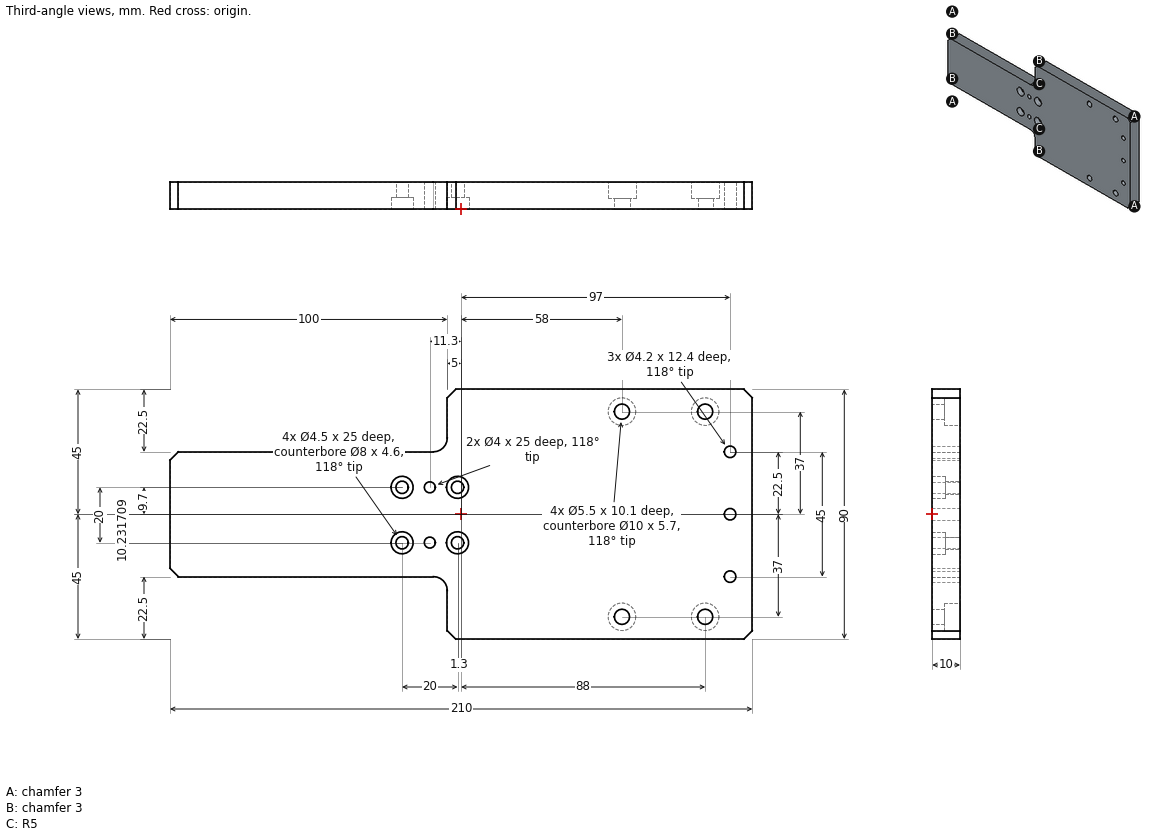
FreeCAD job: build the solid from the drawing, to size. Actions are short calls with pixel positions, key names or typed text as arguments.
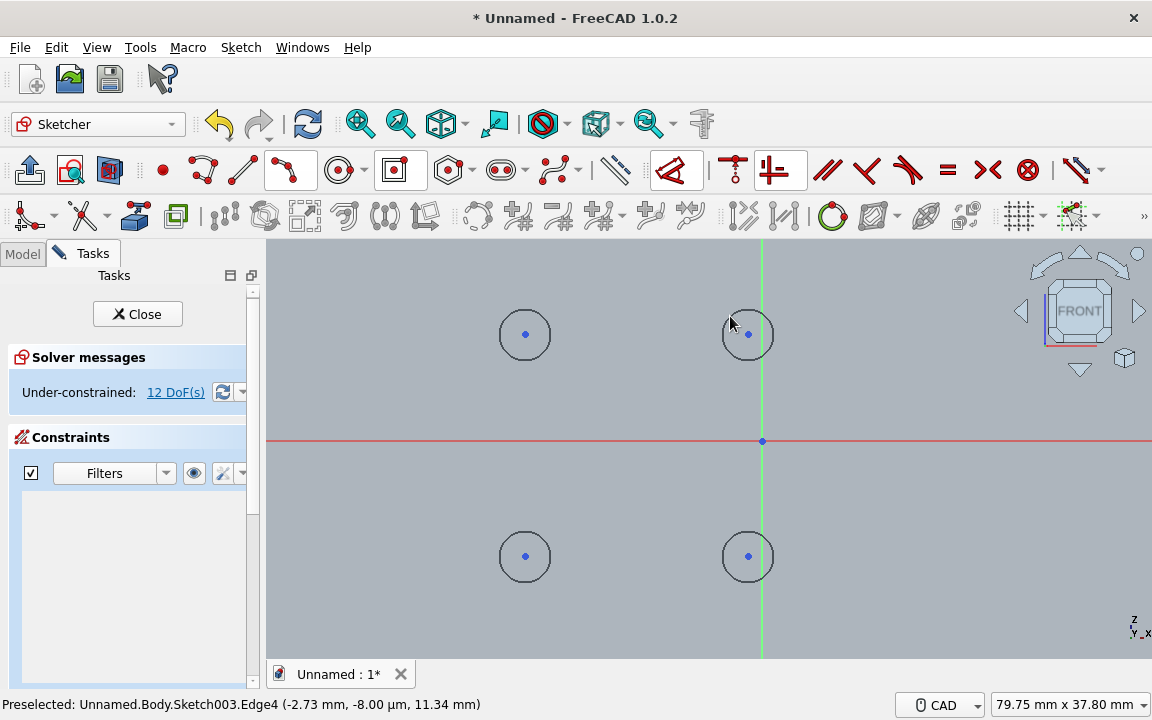
click(543, 539)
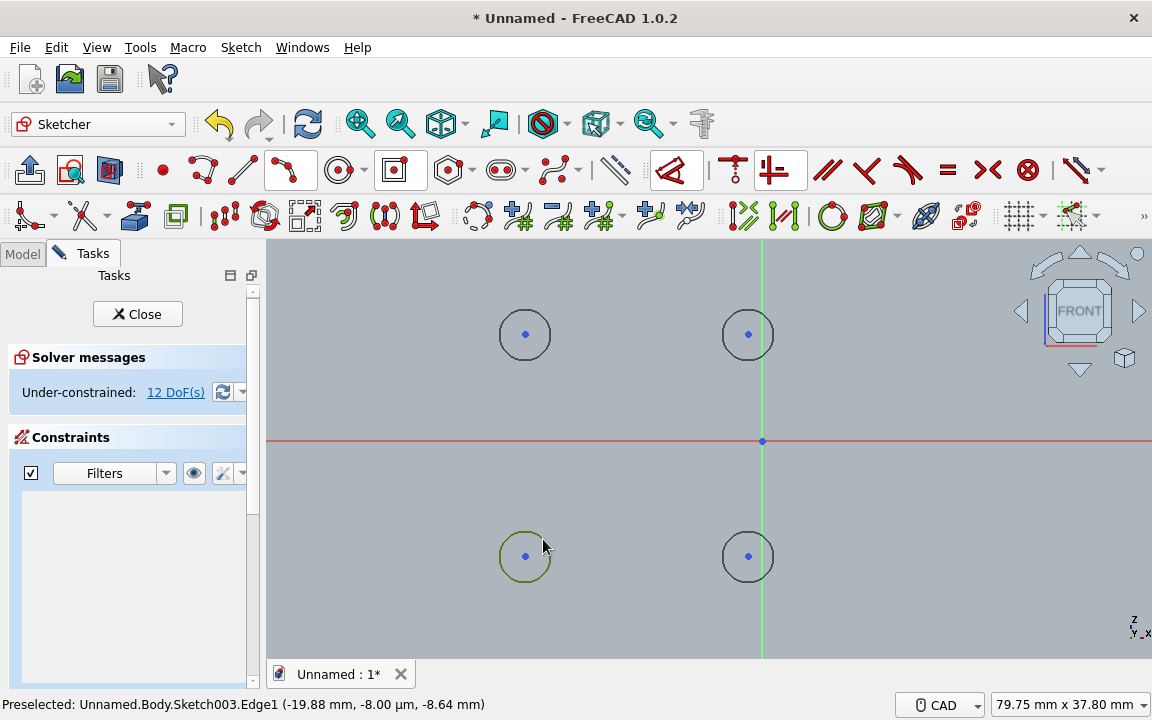
click(543, 317)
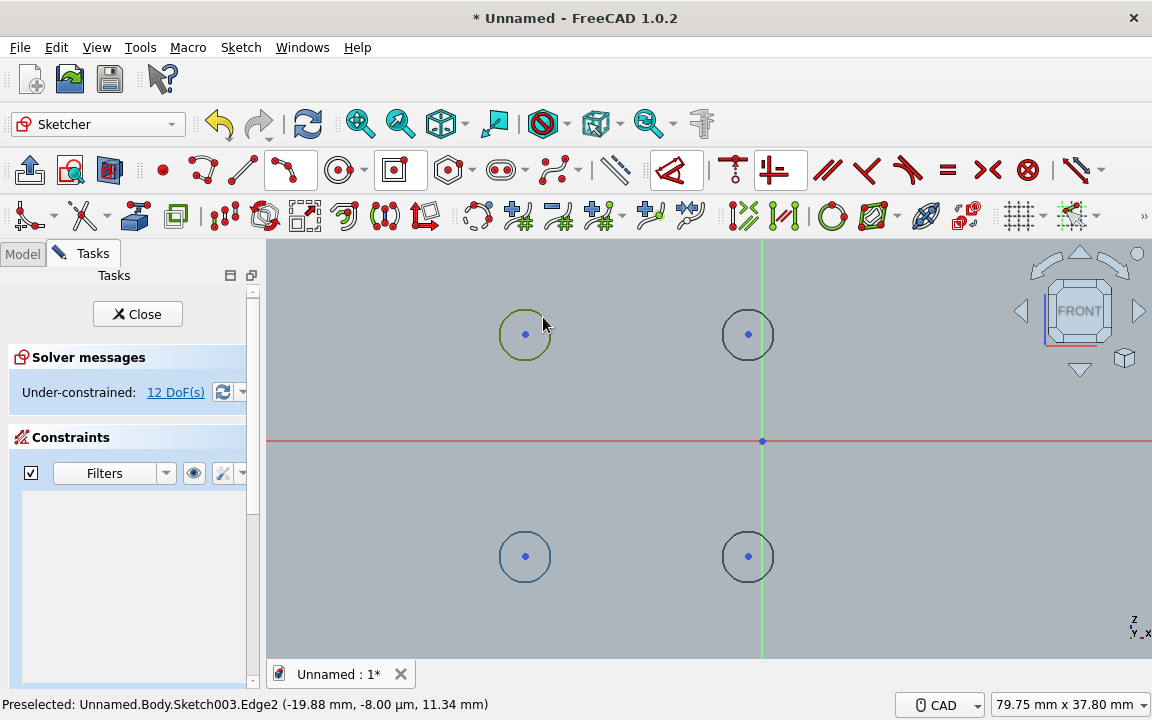
click(766, 539)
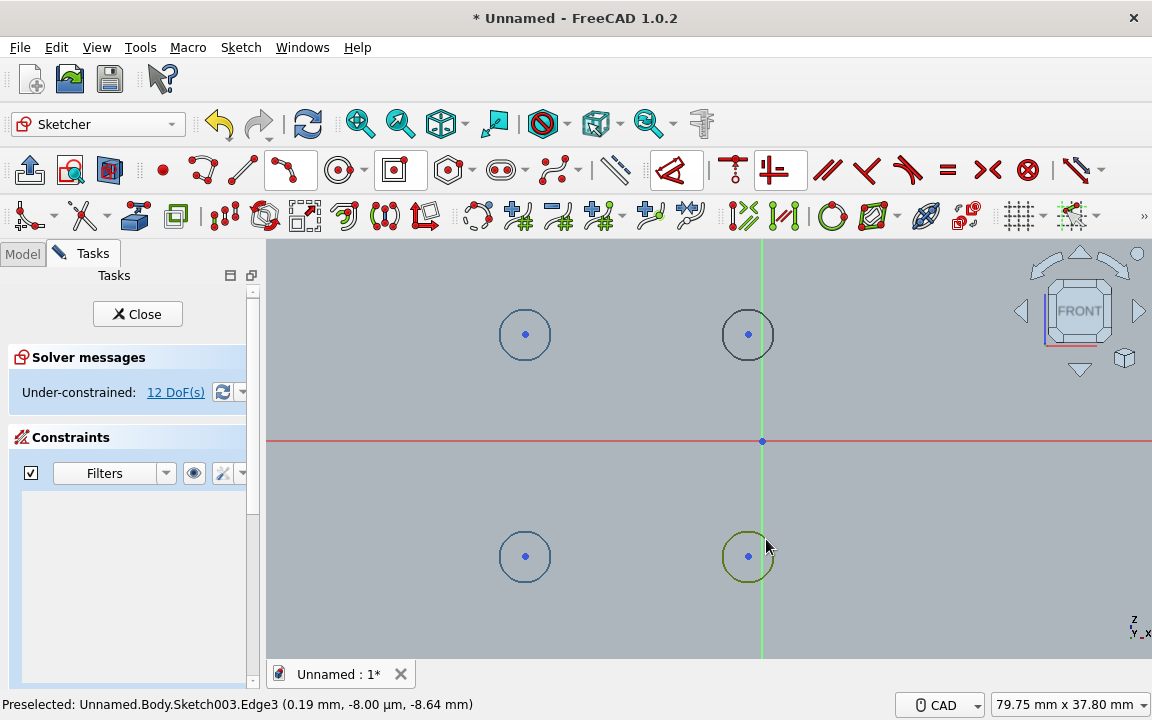
click(766, 317)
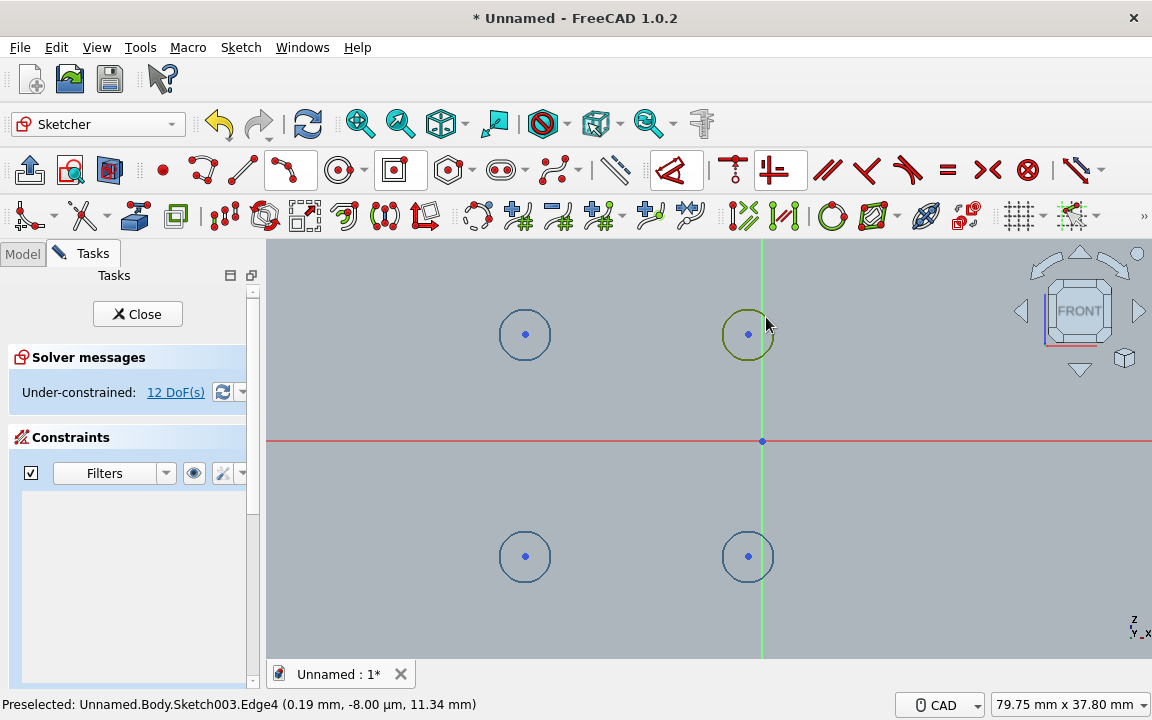
click(948, 170)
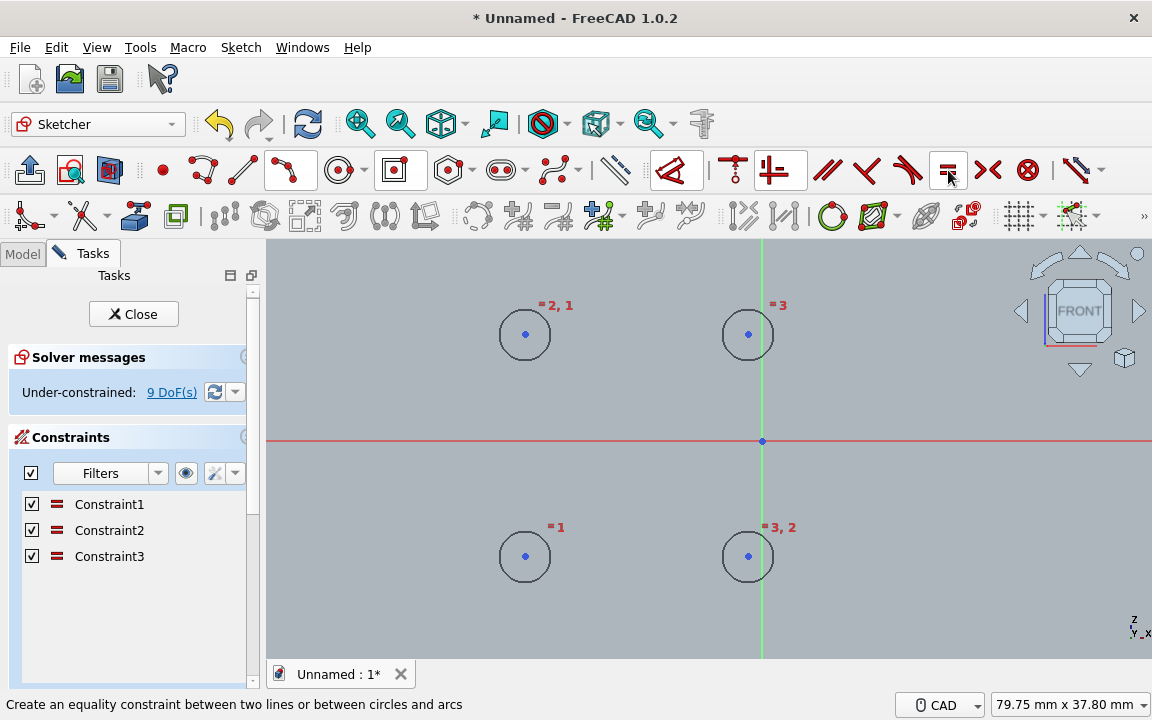
click(525, 557)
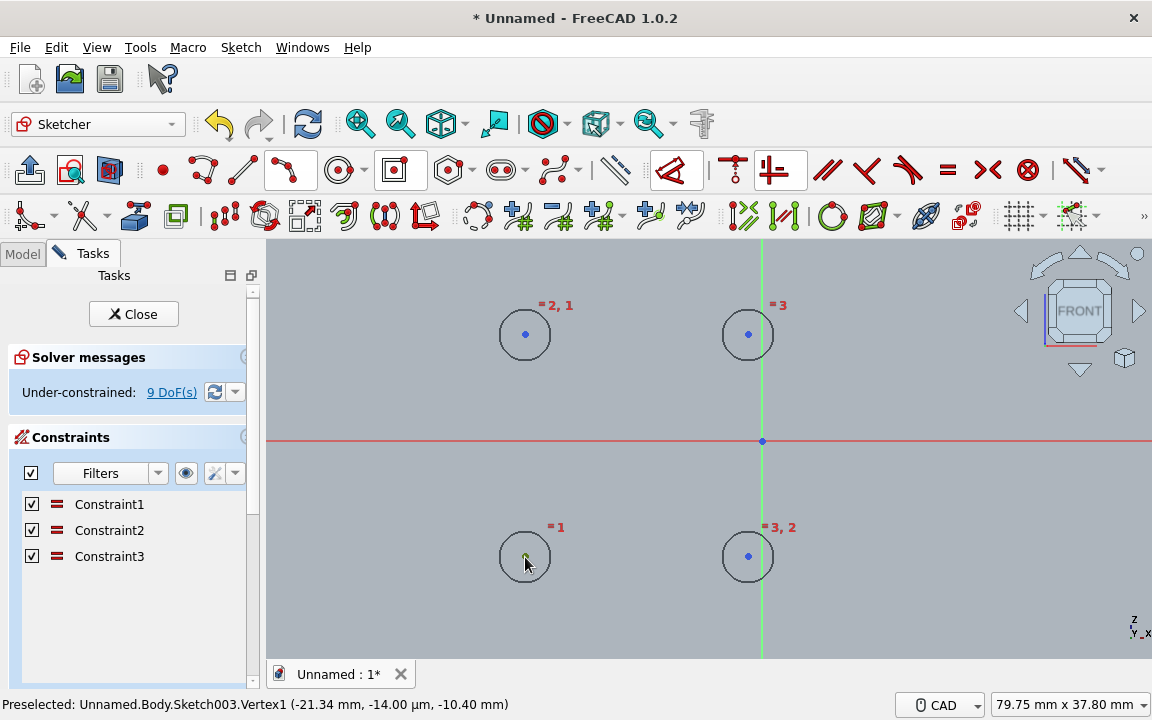
click(525, 335)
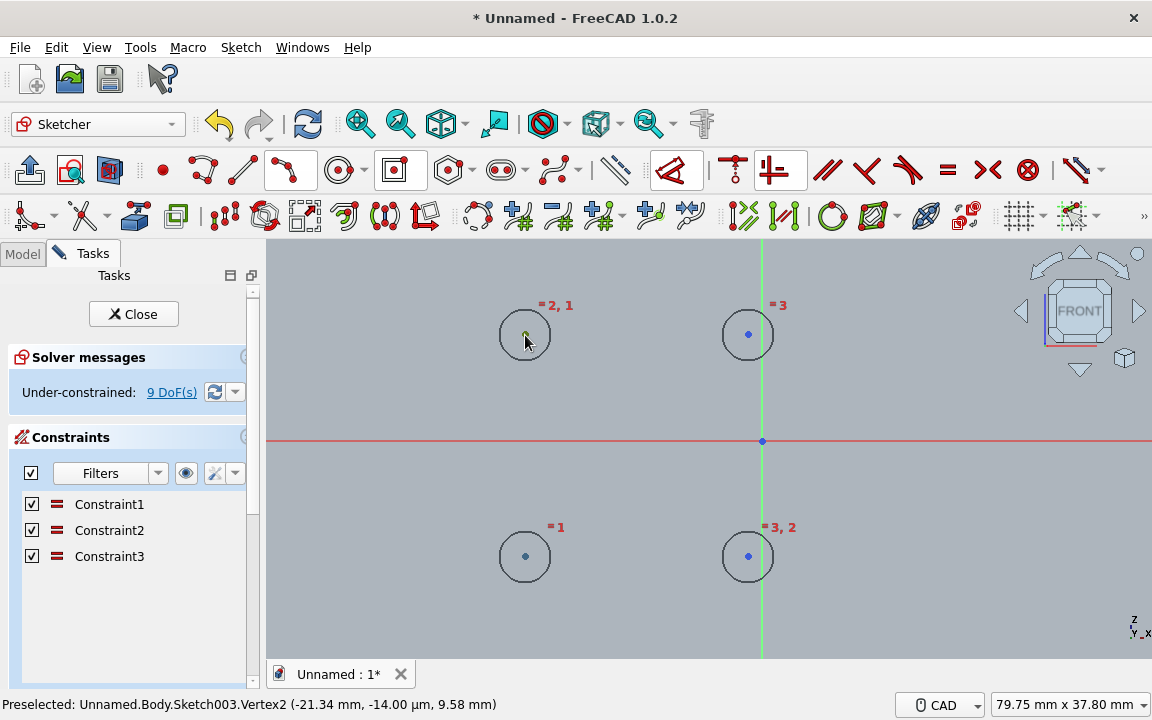
key(v)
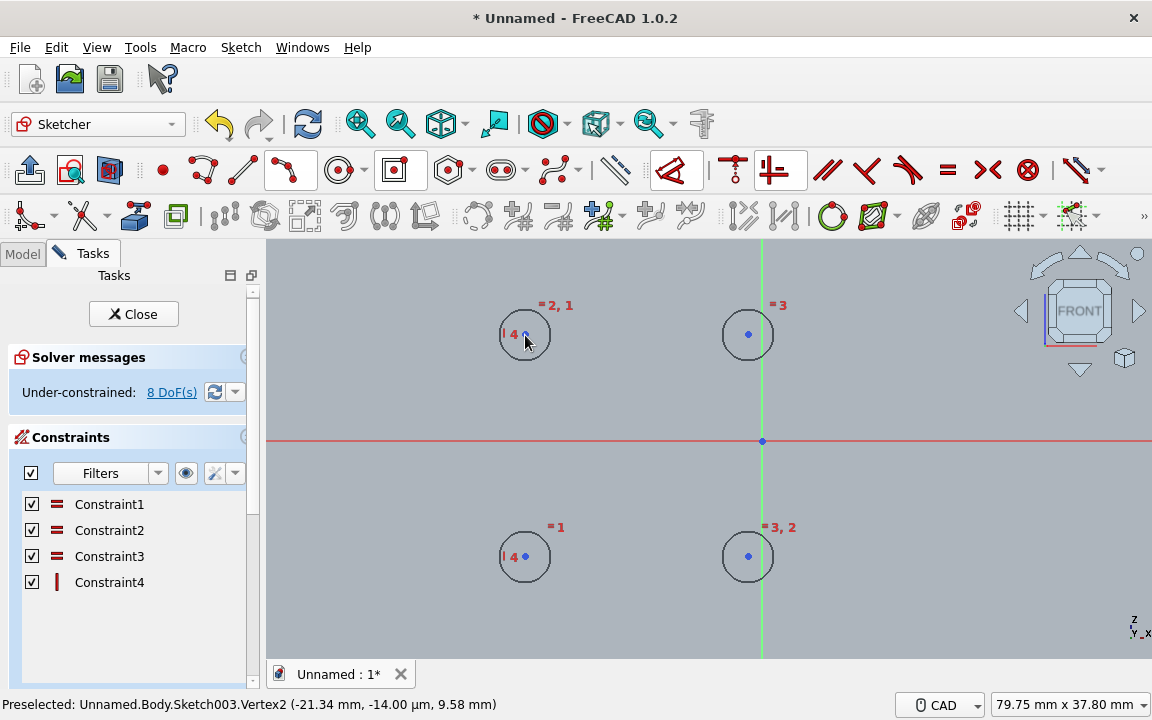
click(525, 557)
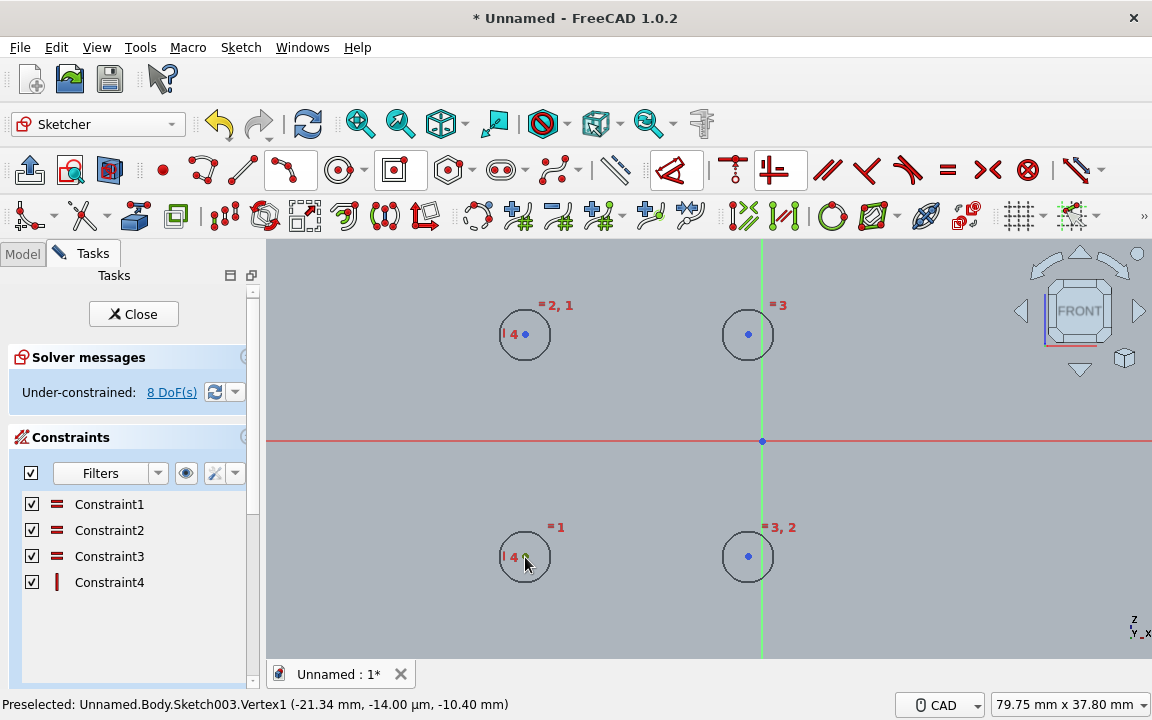
click(748, 557)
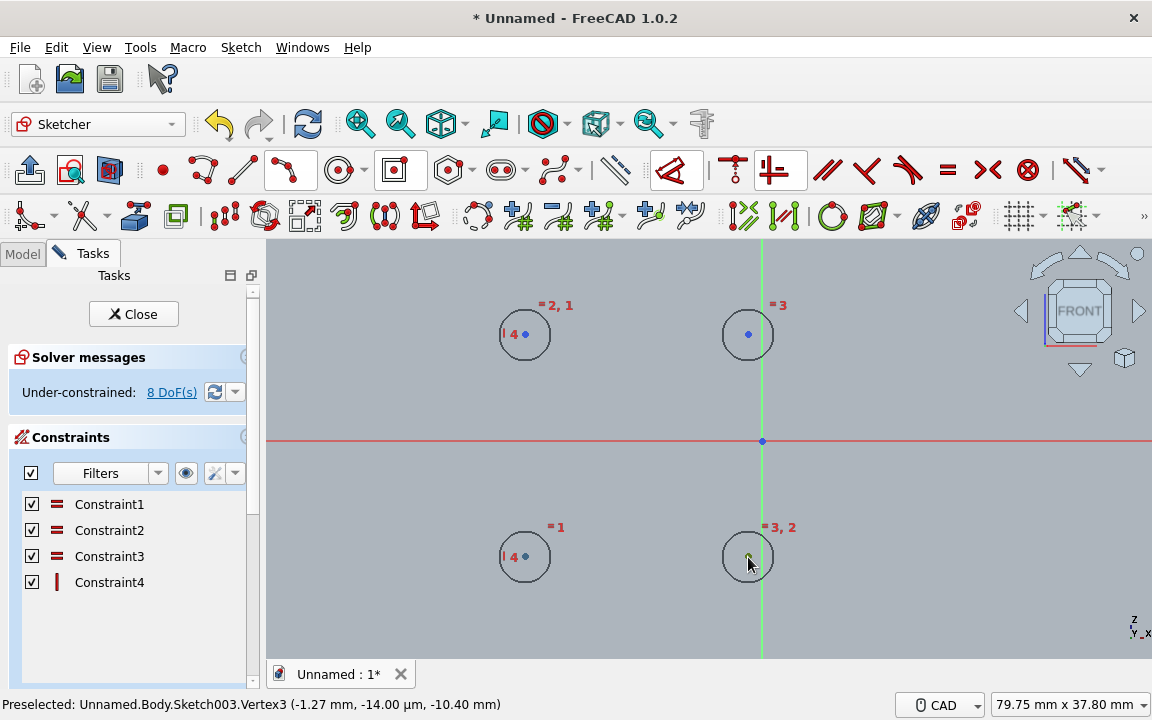
key(h)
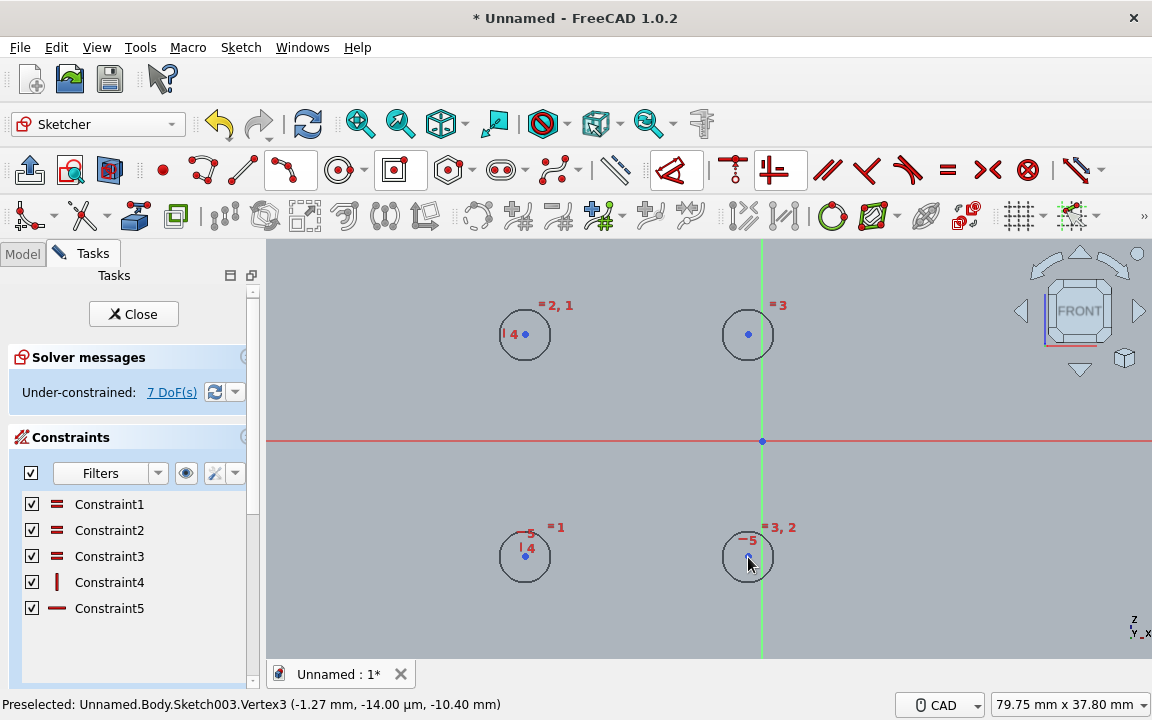
click(748, 557)